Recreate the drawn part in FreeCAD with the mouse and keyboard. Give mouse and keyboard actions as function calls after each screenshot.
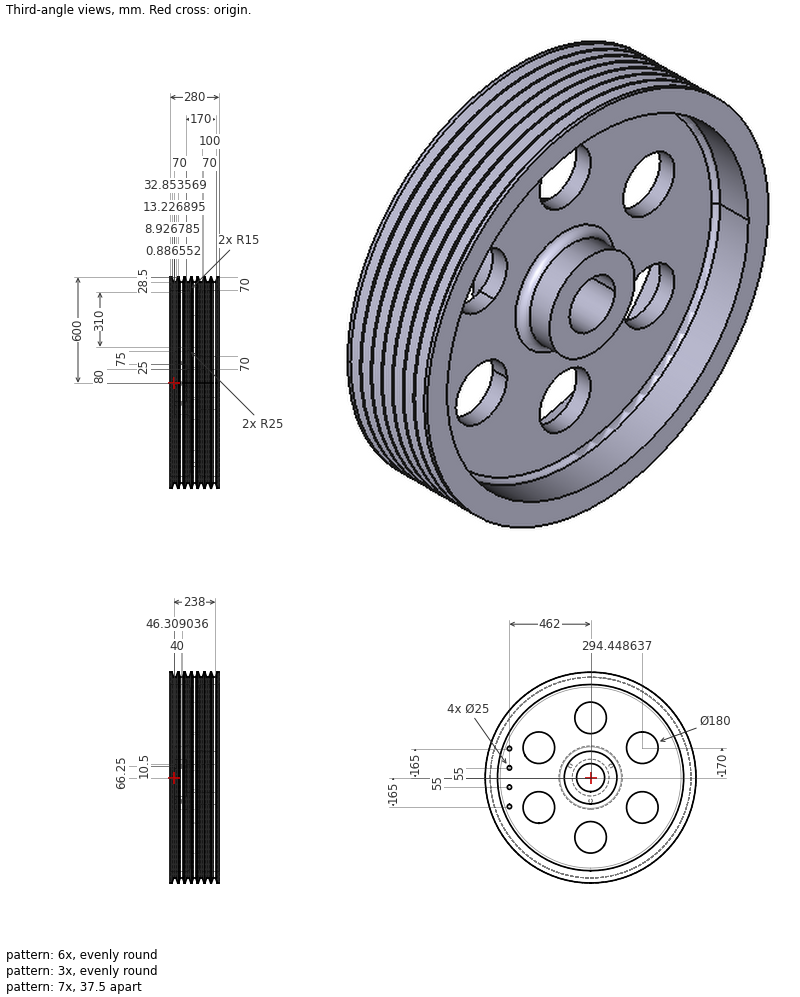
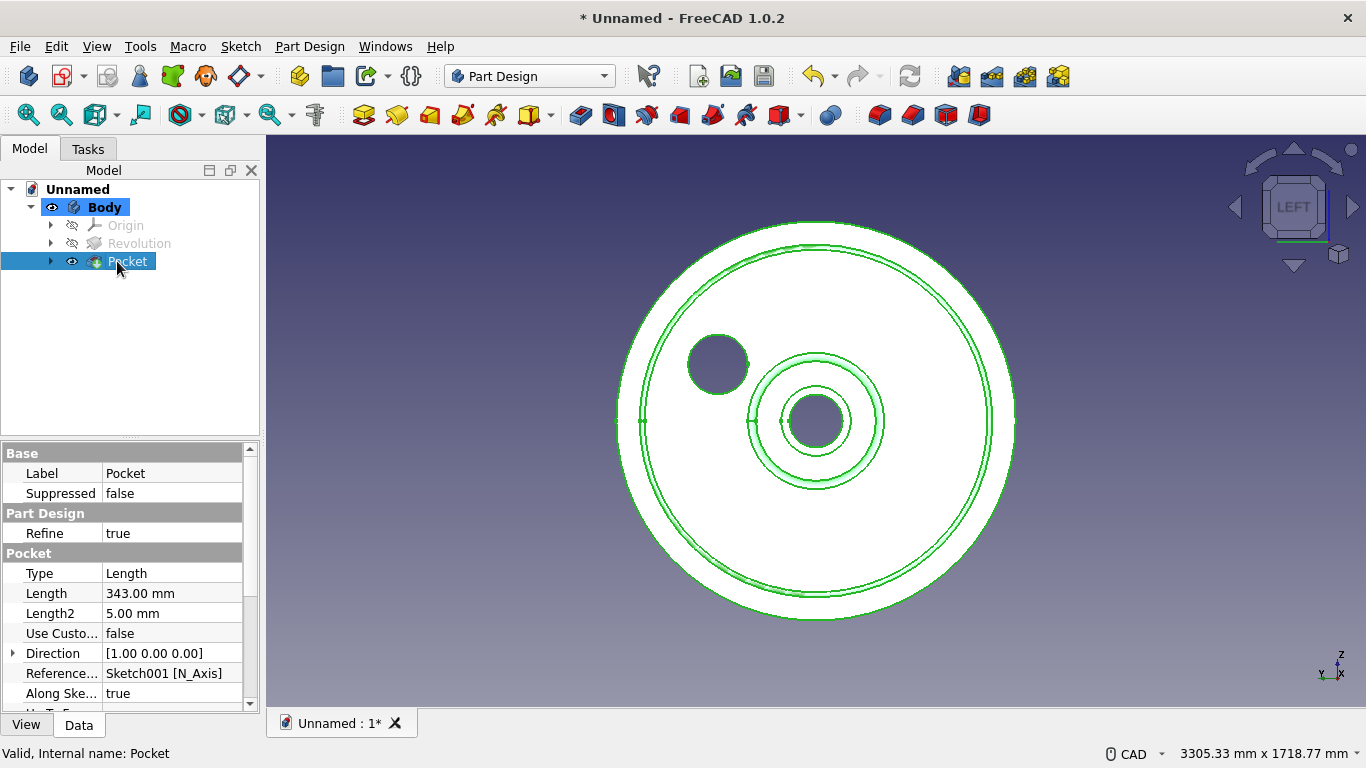
click(1025, 76)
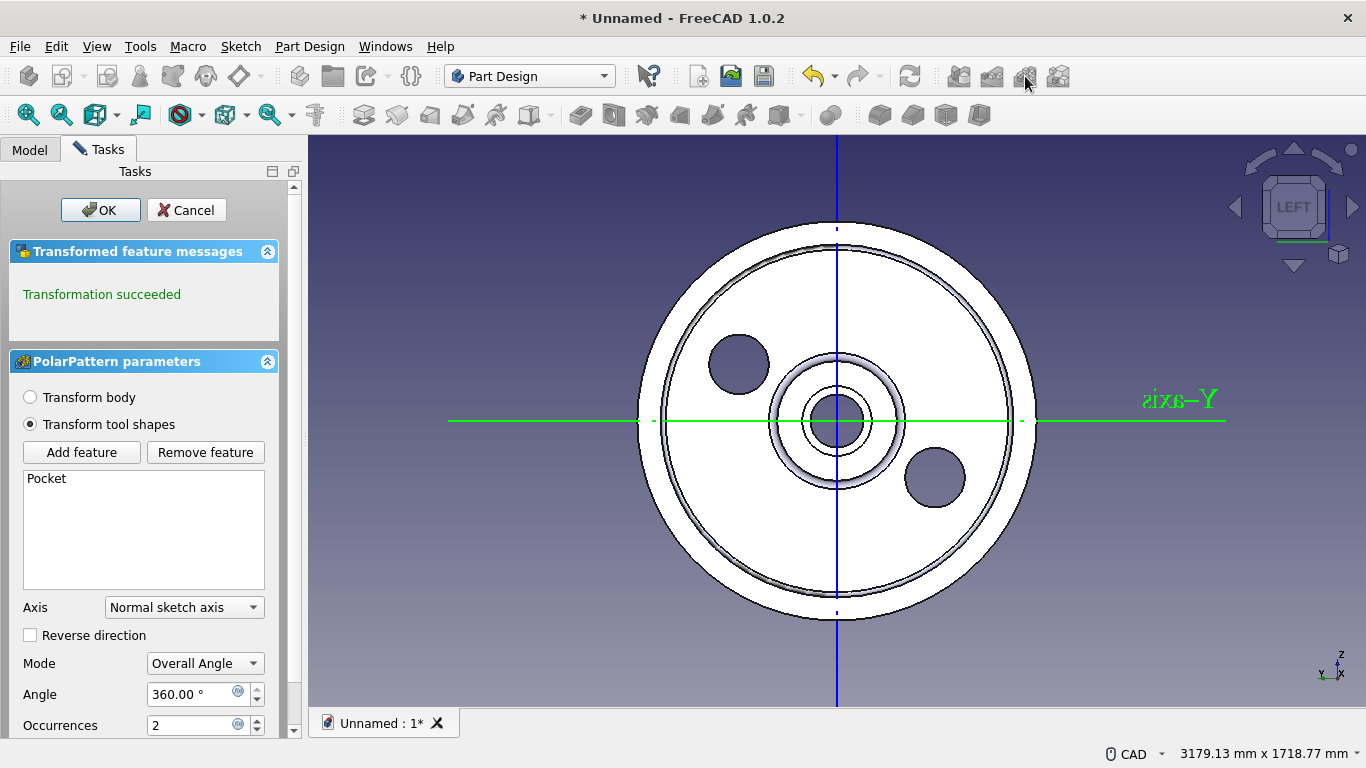
click(185, 608)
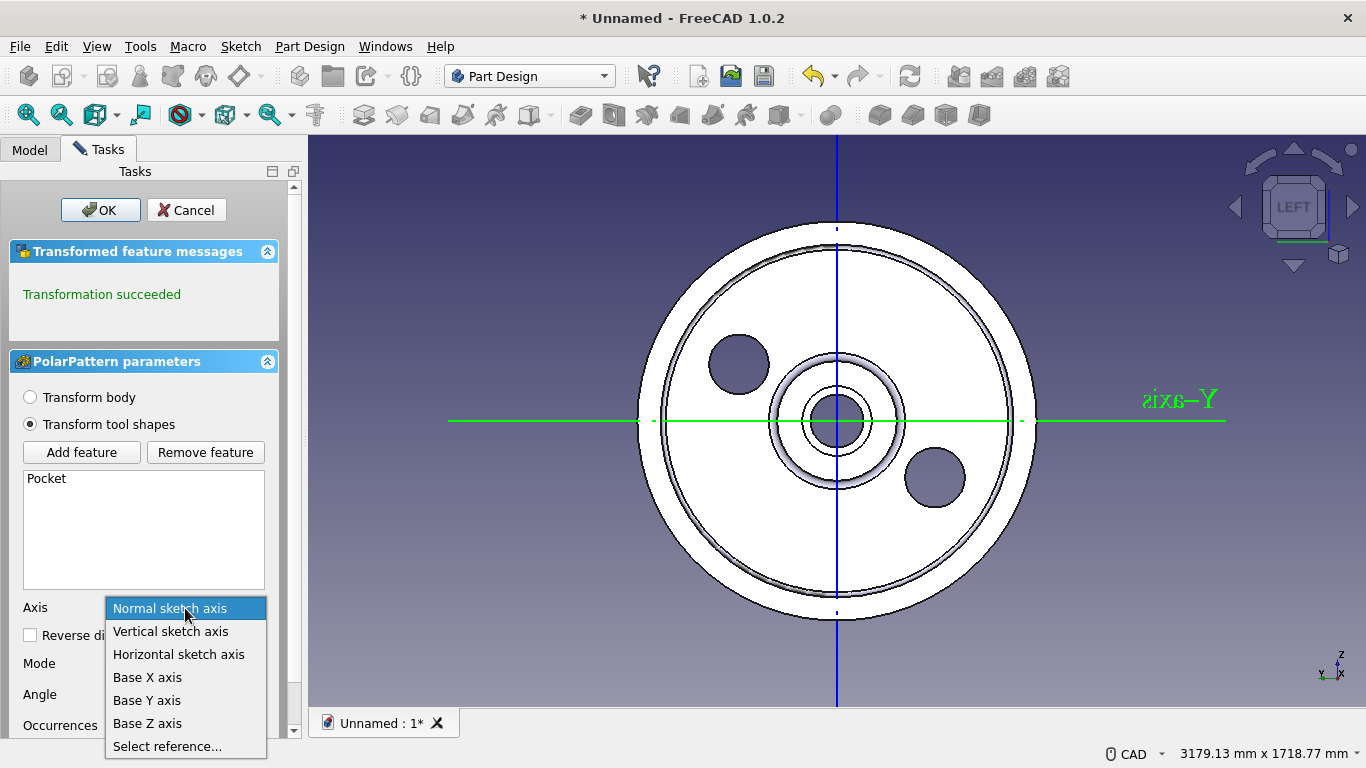
click(184, 678)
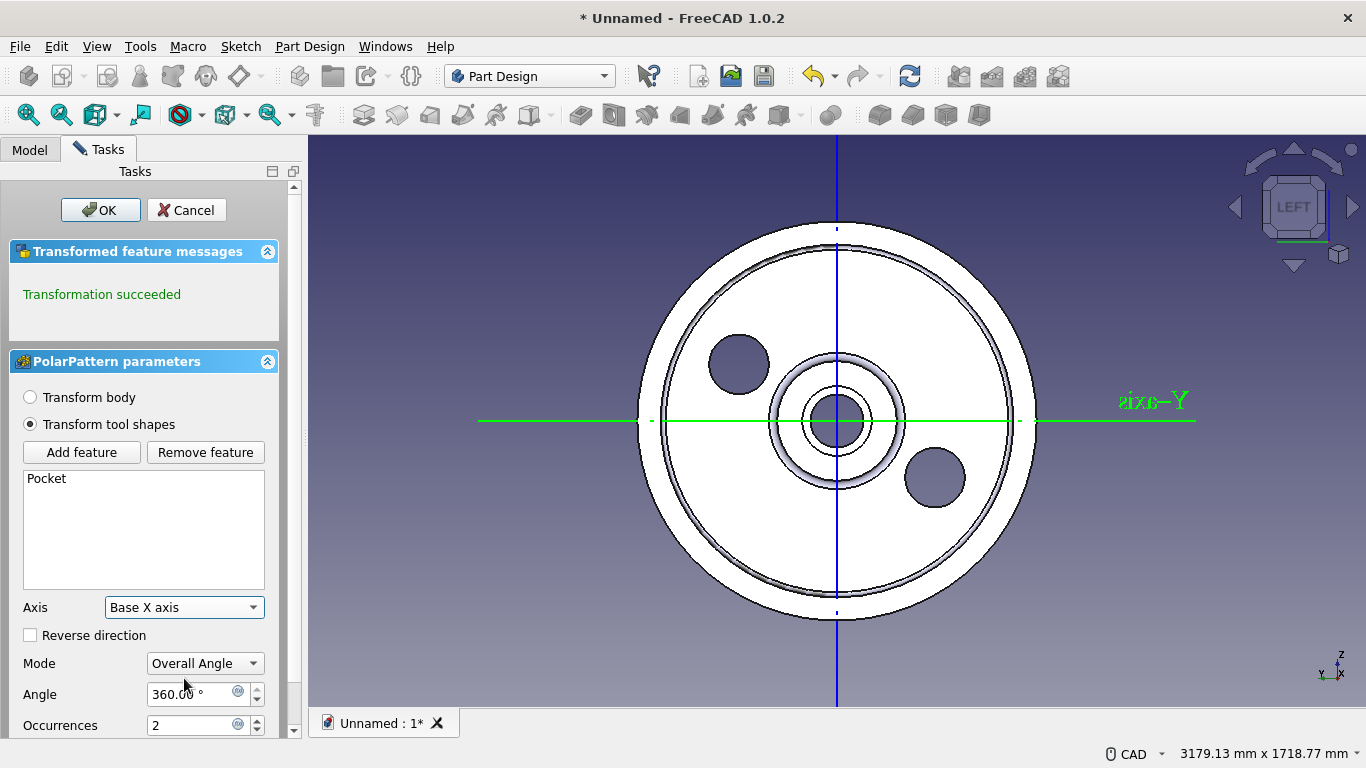
triple_click(199, 726)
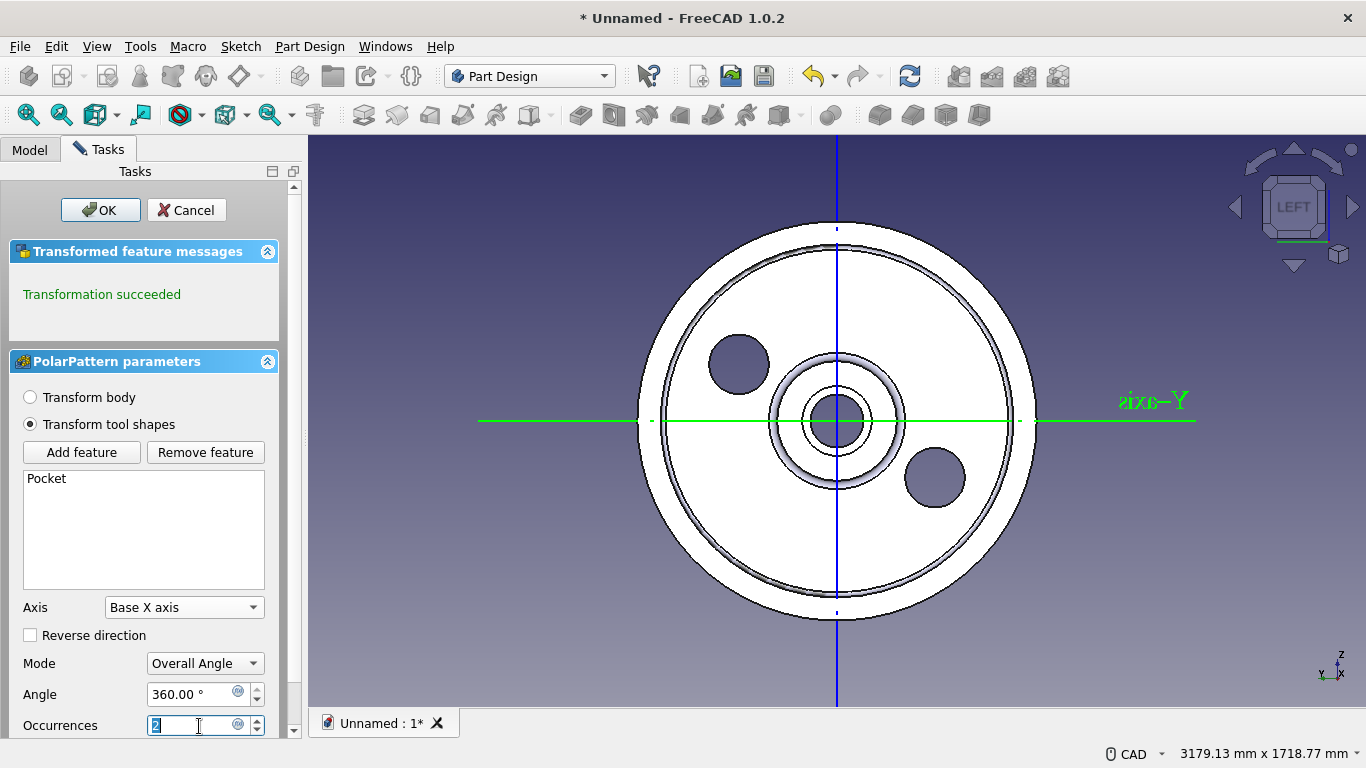
text(6)
key(Tab)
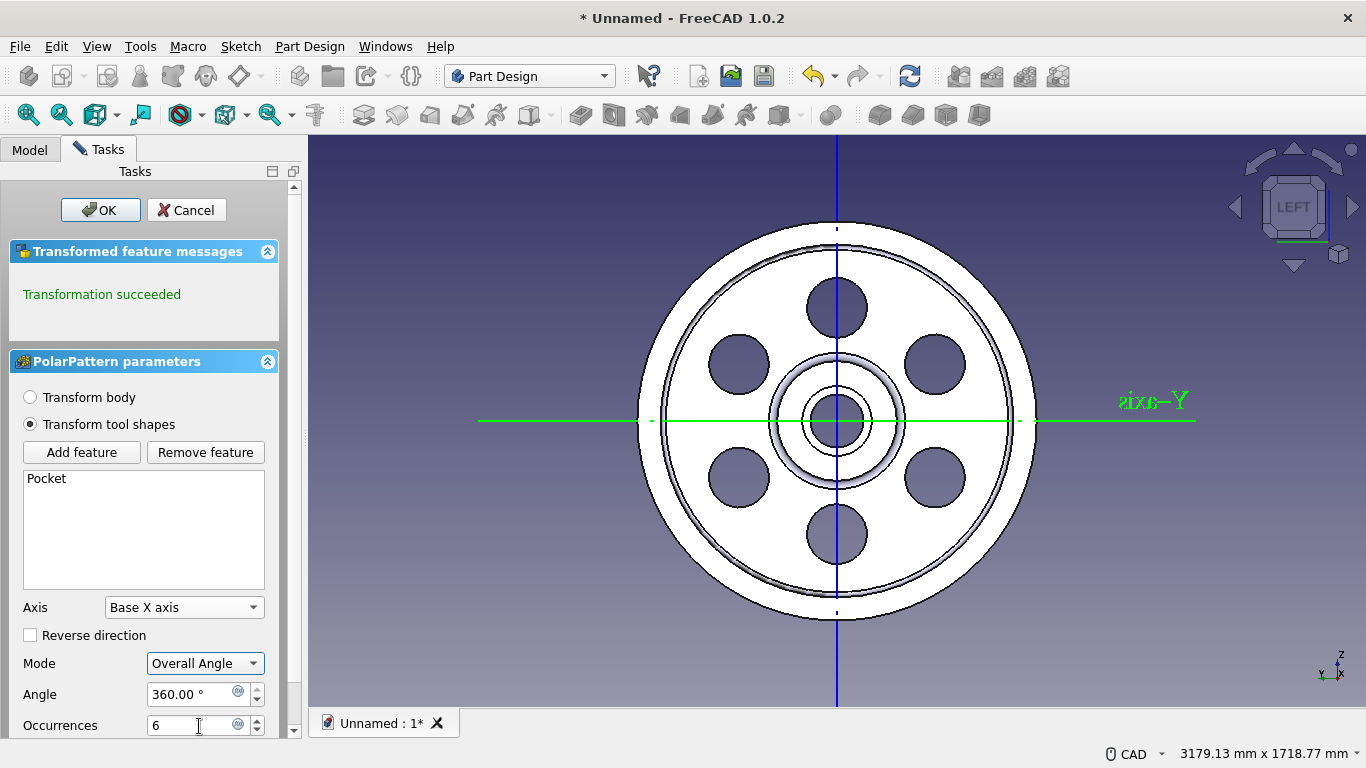
click(101, 210)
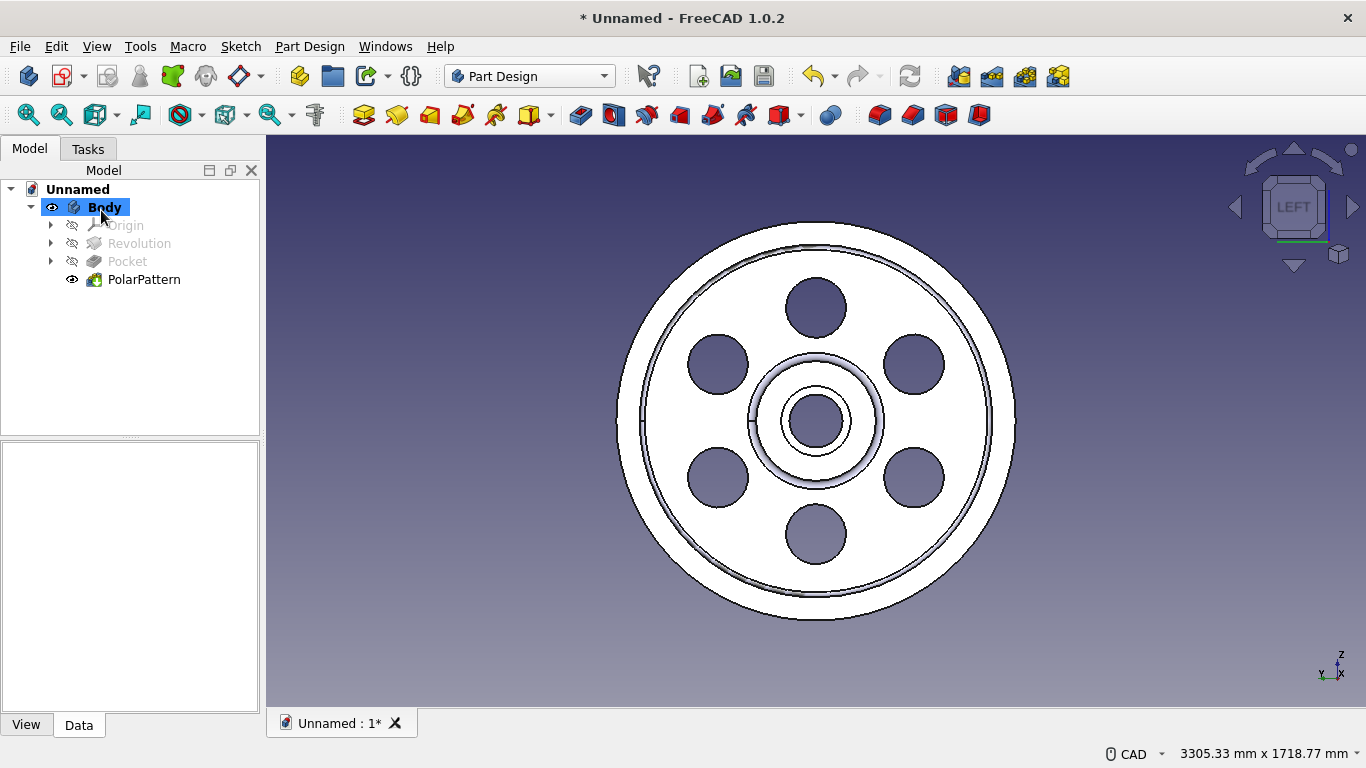
click(51, 225)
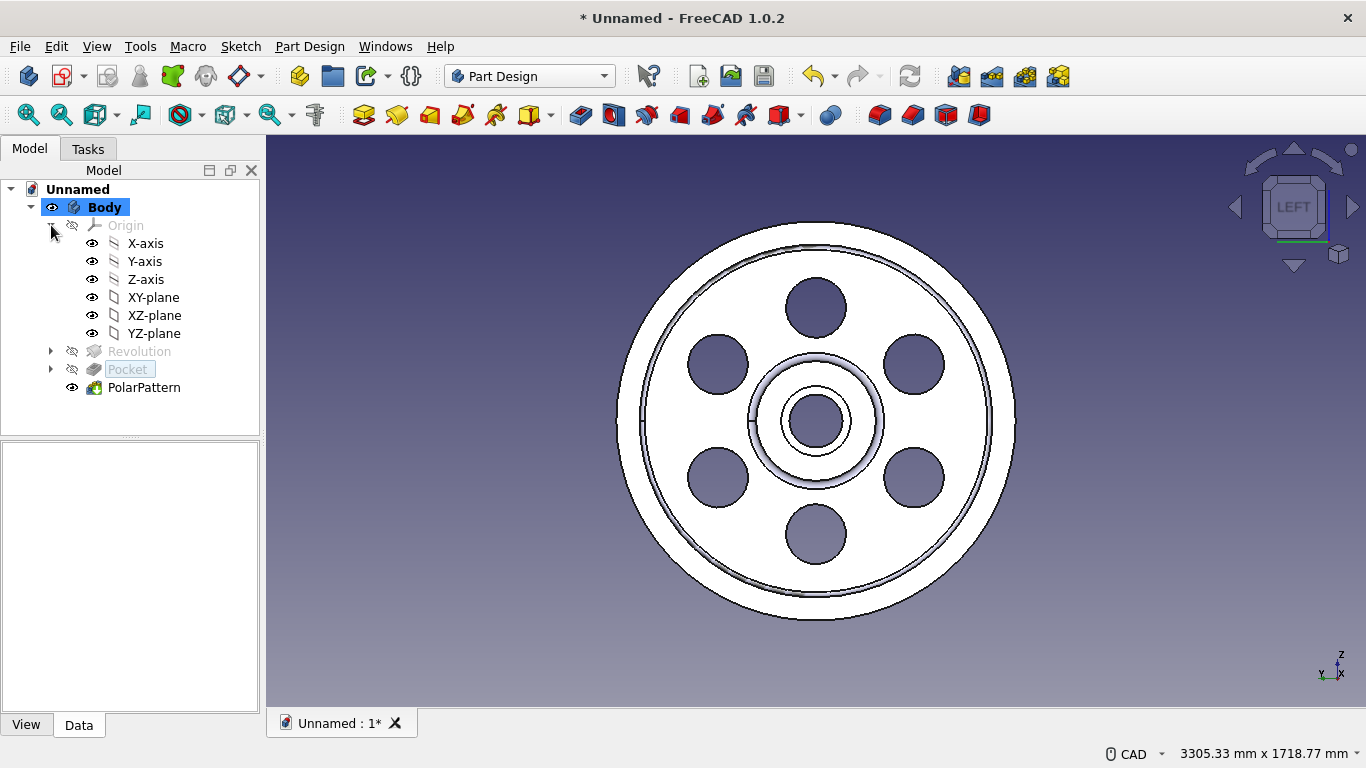
click(137, 315)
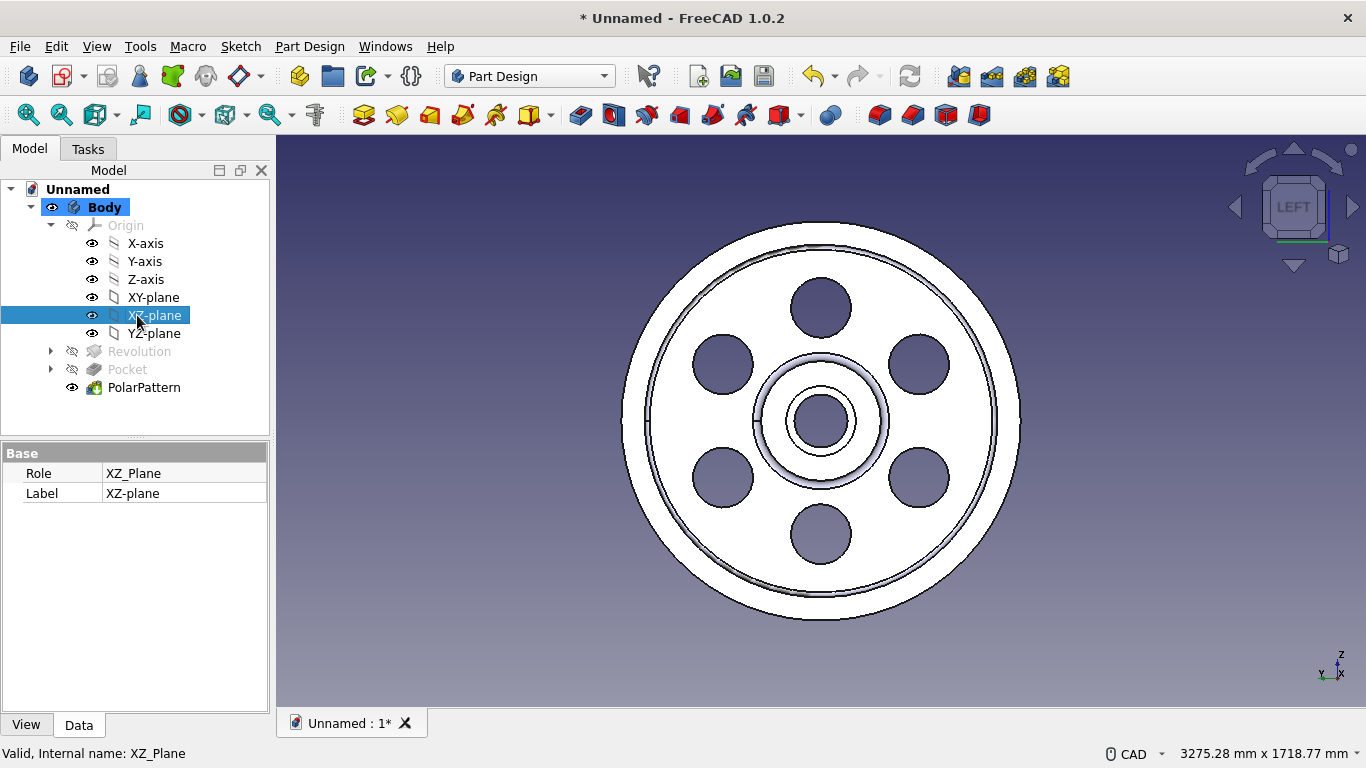
click(238, 76)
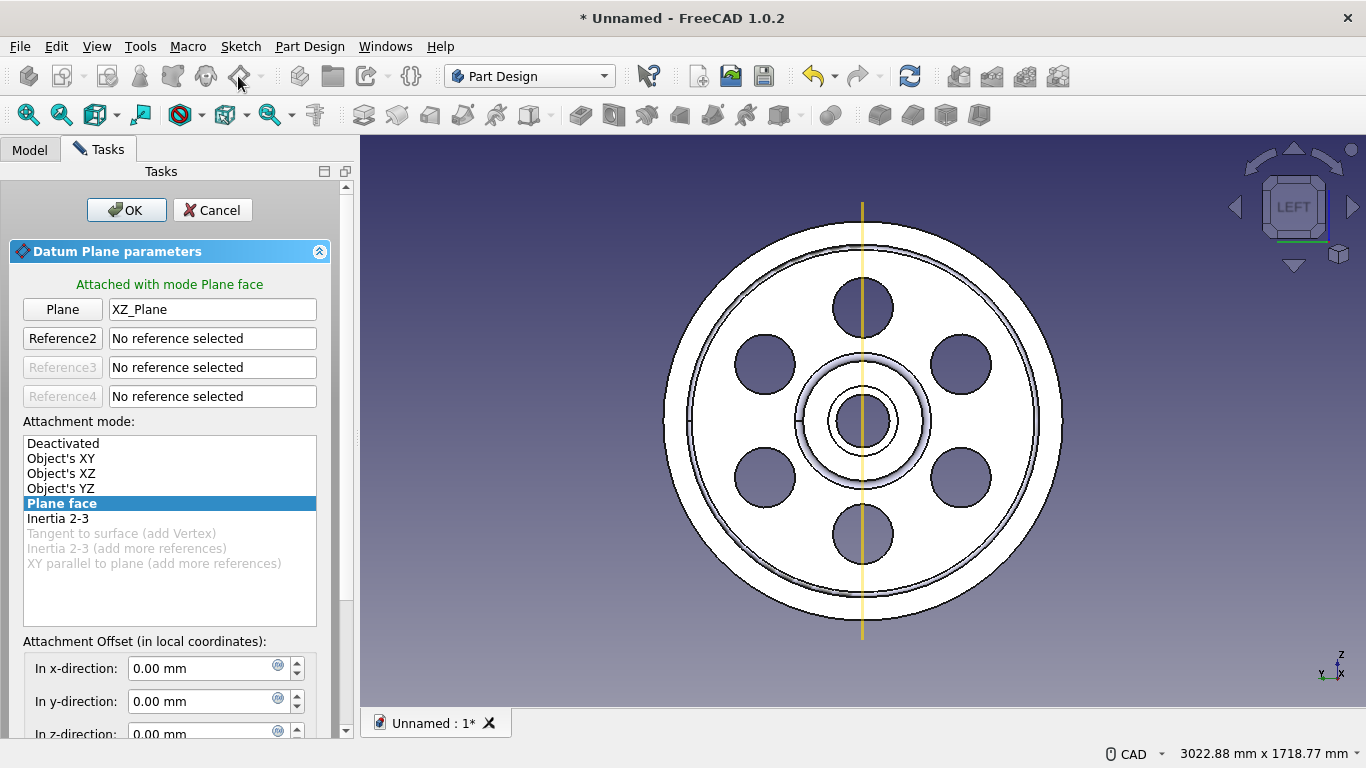
scroll(346, 460, down, 2)